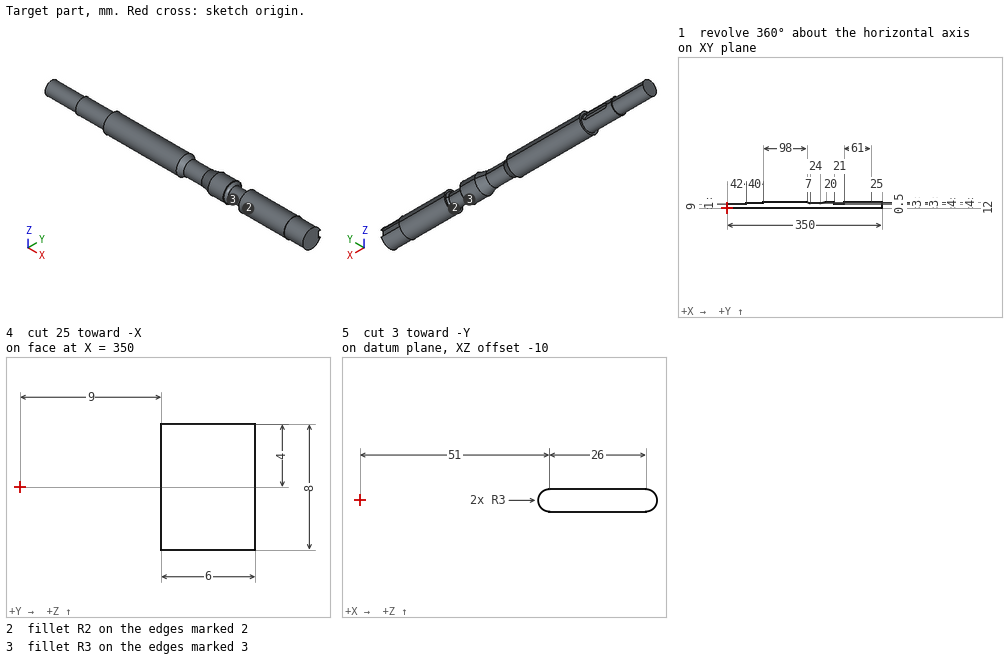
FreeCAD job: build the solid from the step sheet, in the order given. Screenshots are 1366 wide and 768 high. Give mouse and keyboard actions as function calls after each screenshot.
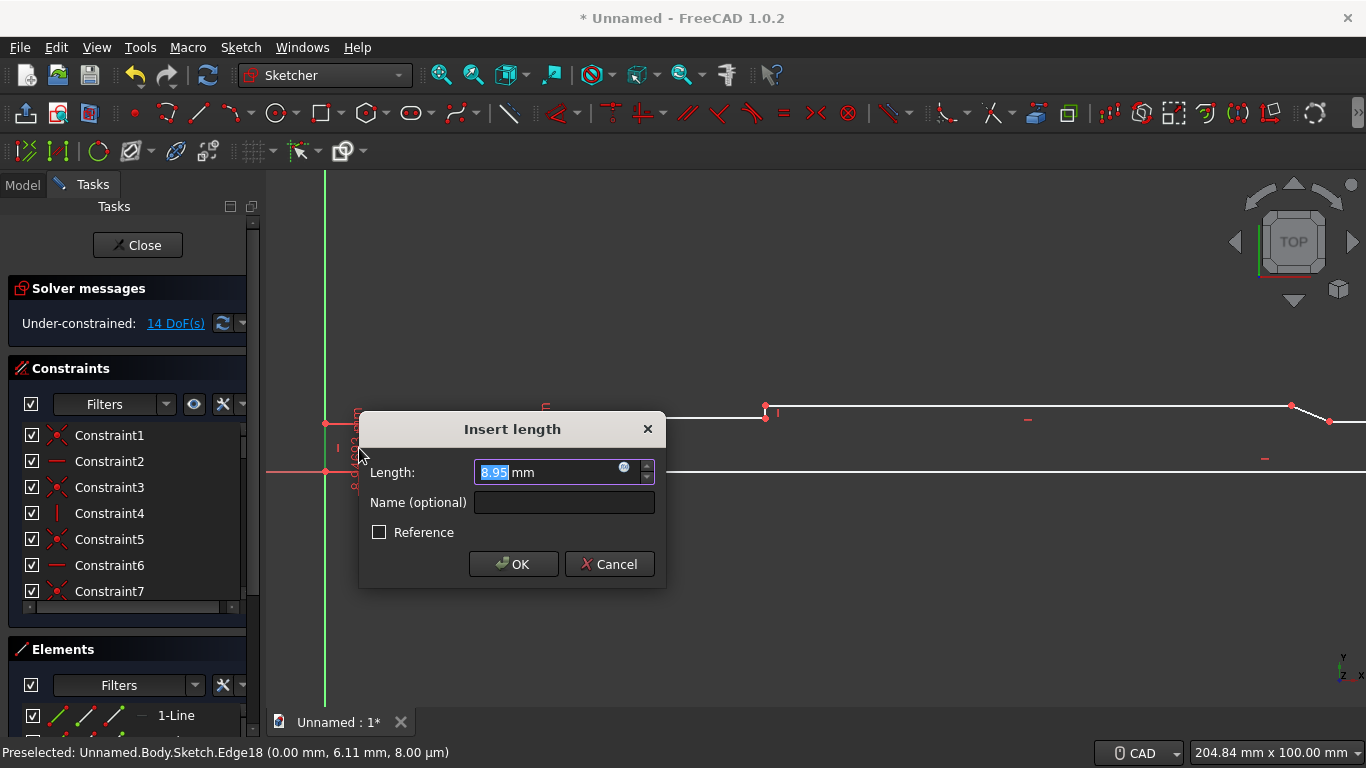
text(9)
key(Return)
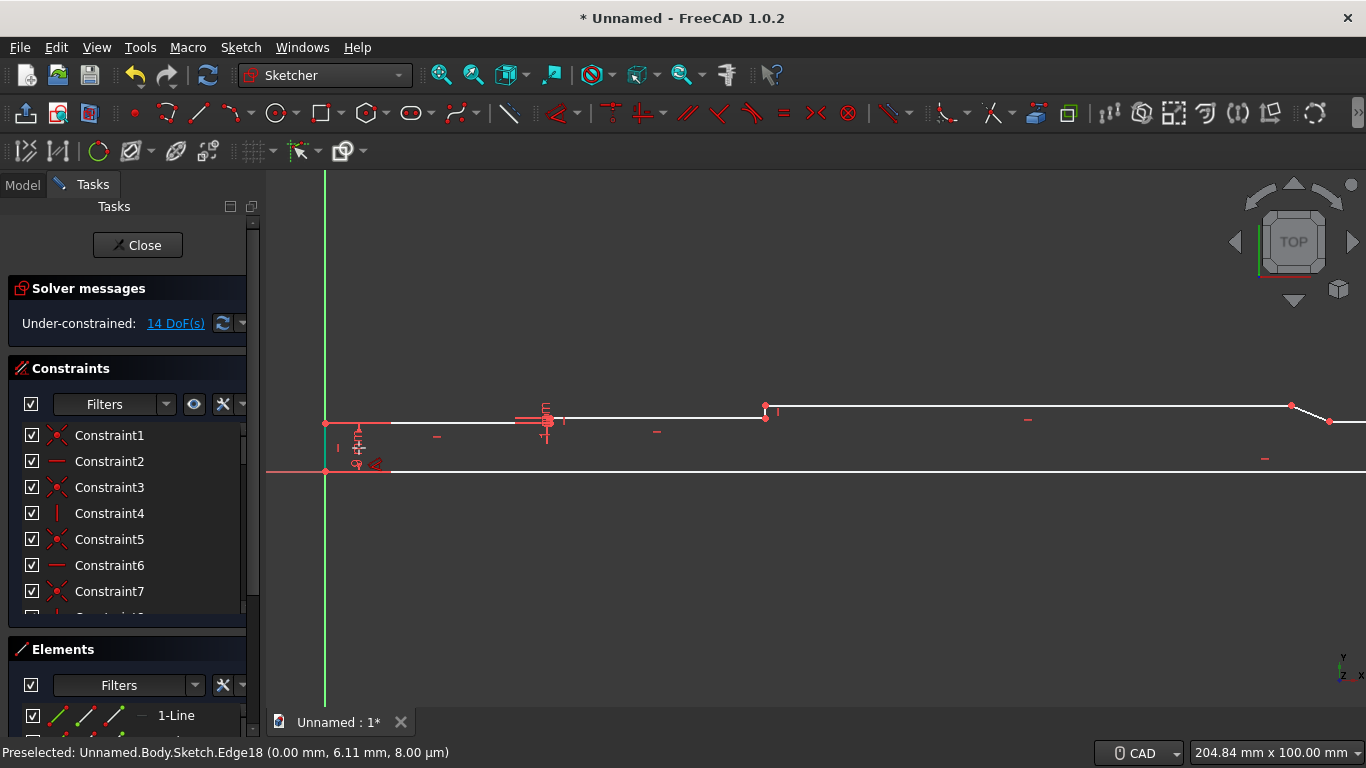
scroll(446, 439, down, 5)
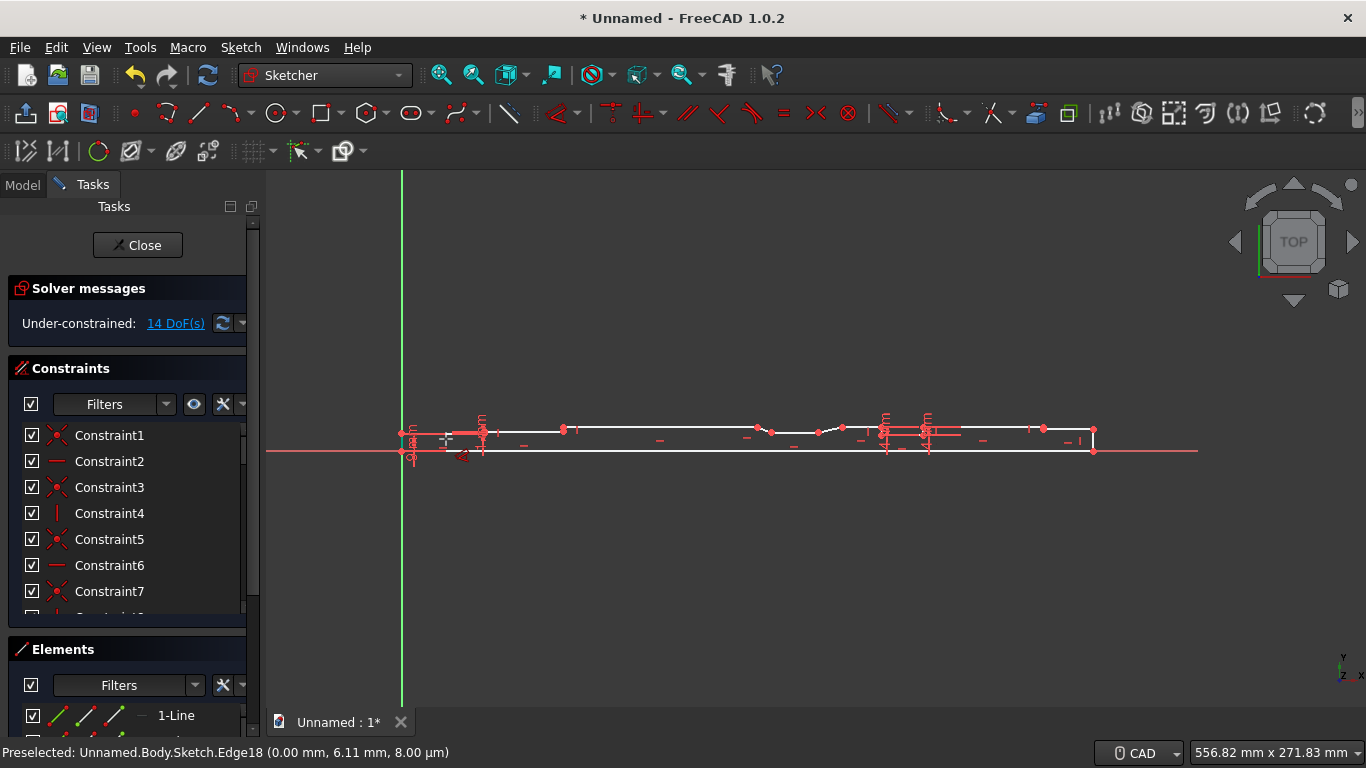
scroll(1093, 445, up, 4)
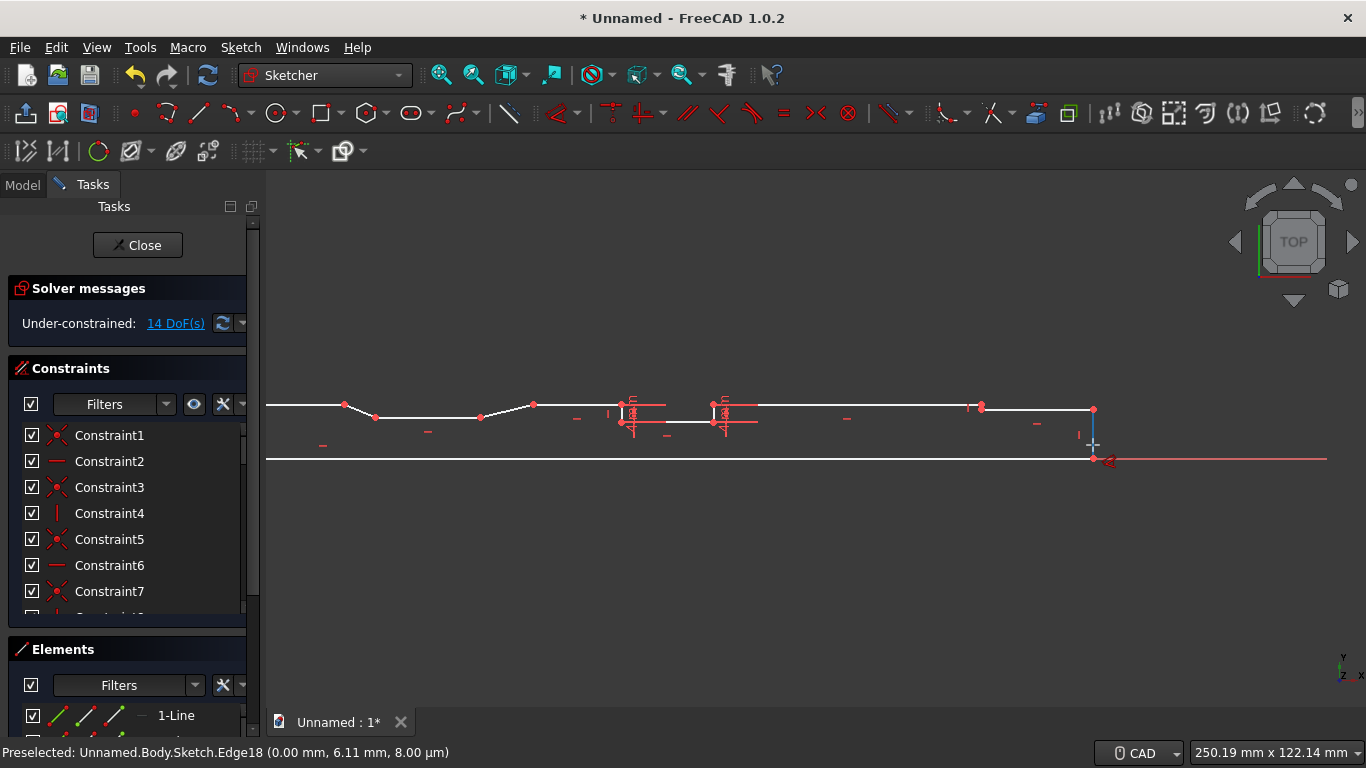
click(1093, 444)
click(1127, 434)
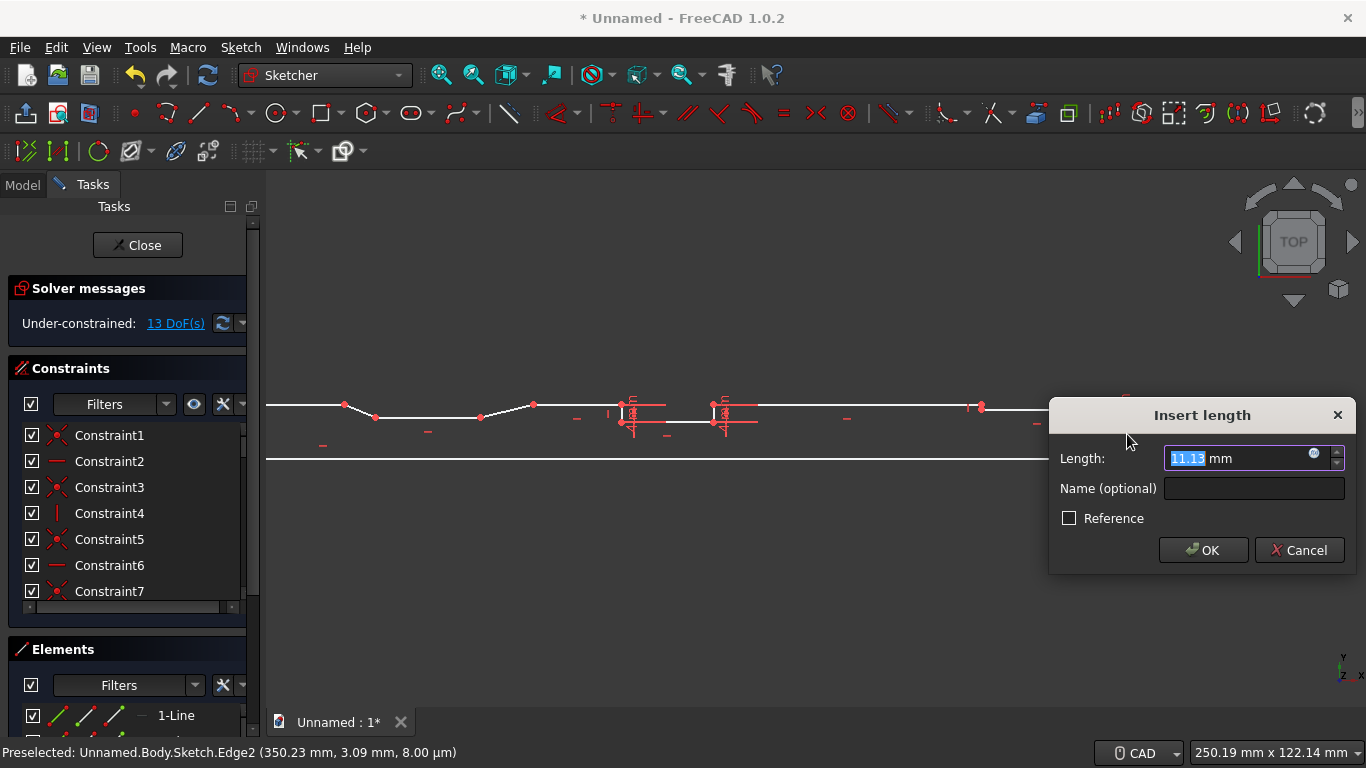
text(12)
key(Return)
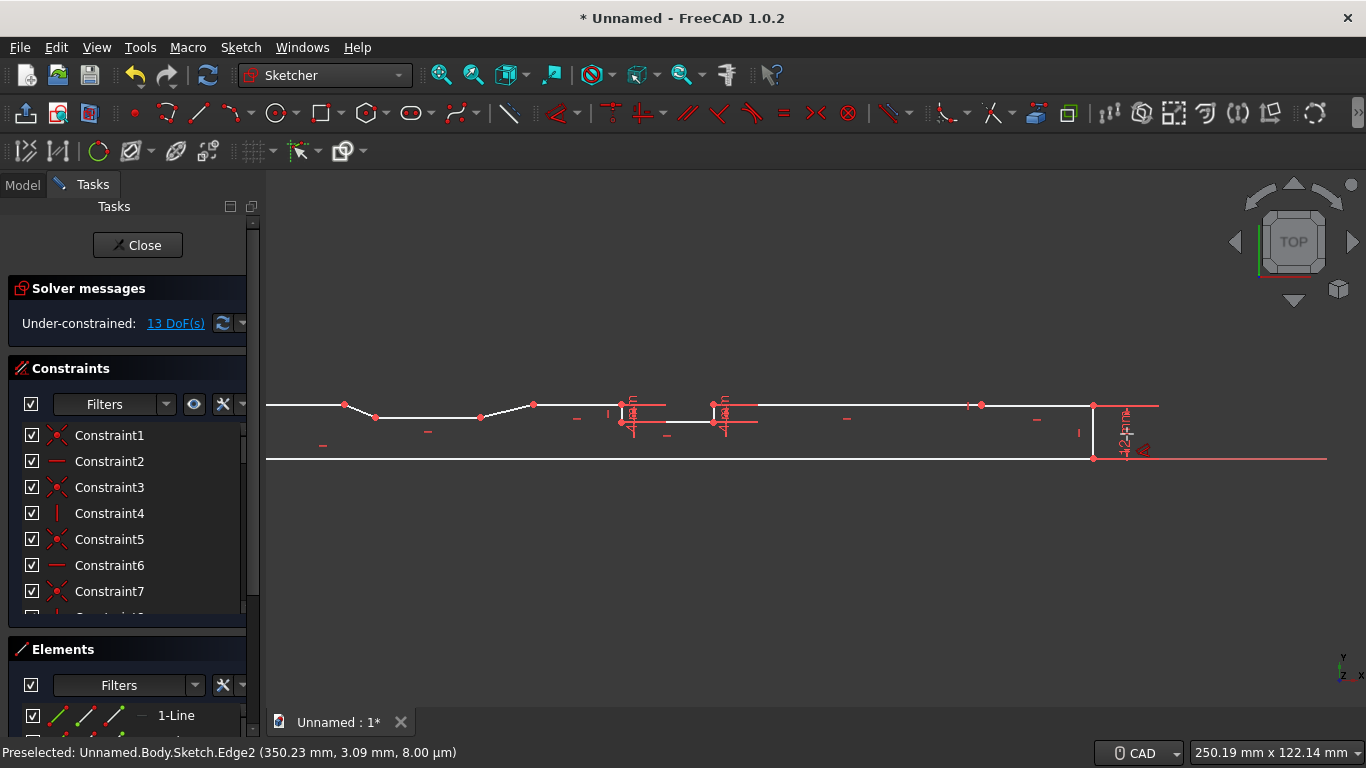
click(1060, 406)
click(1037, 372)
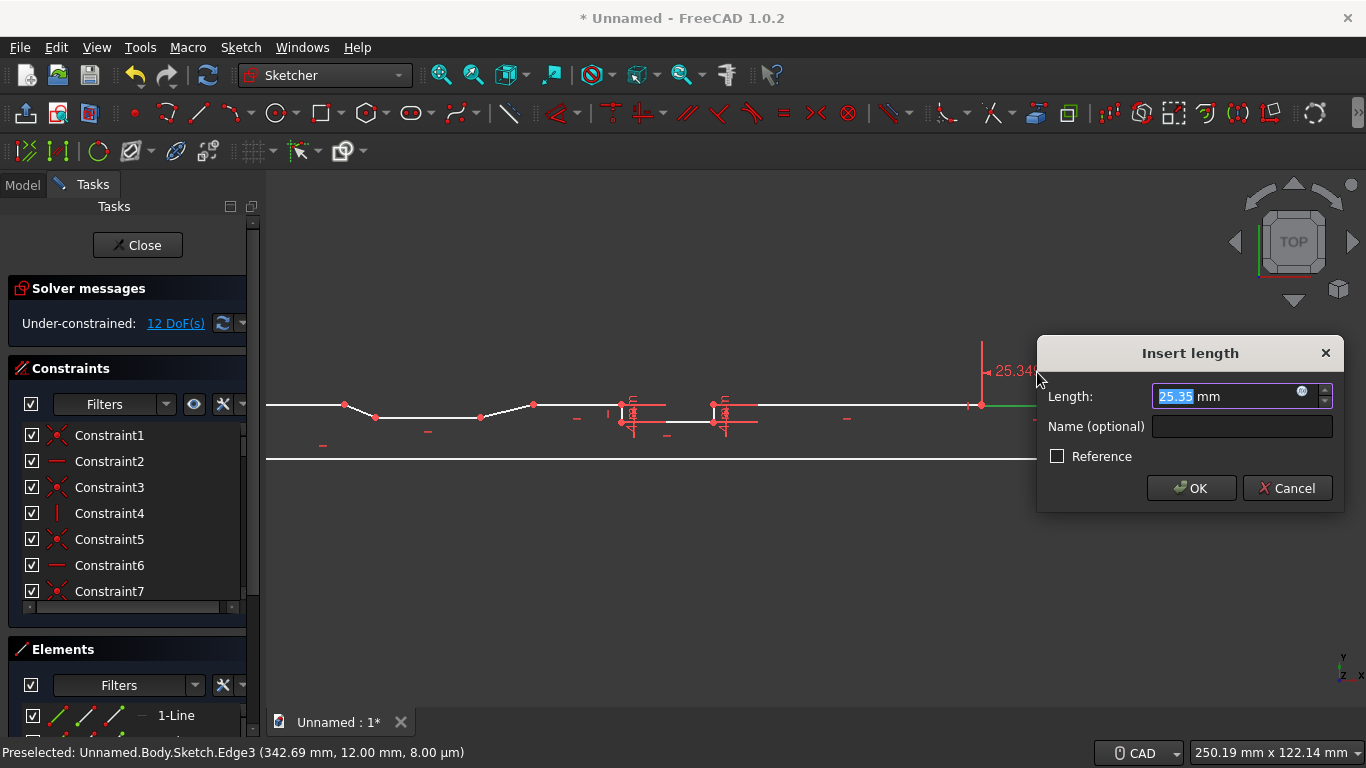
text(25)
key(Return)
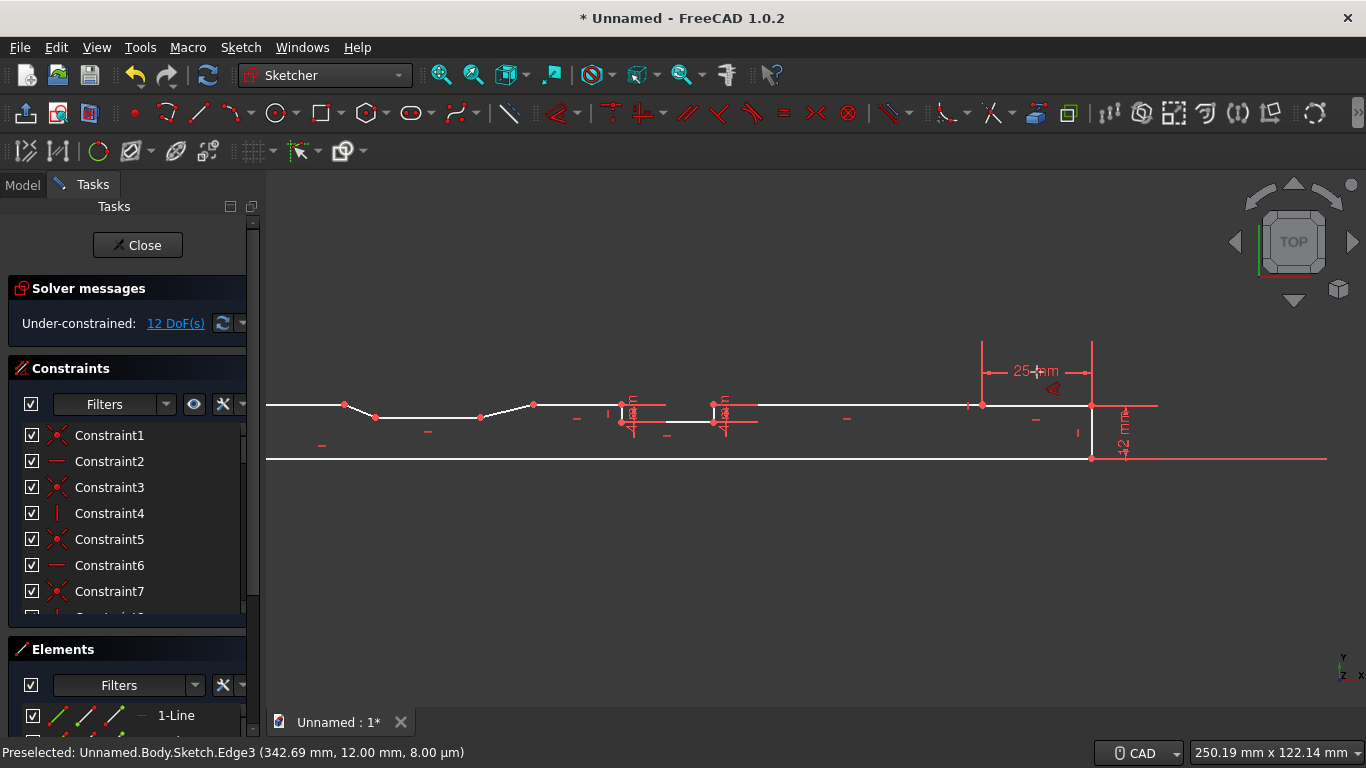
click(902, 405)
click(848, 371)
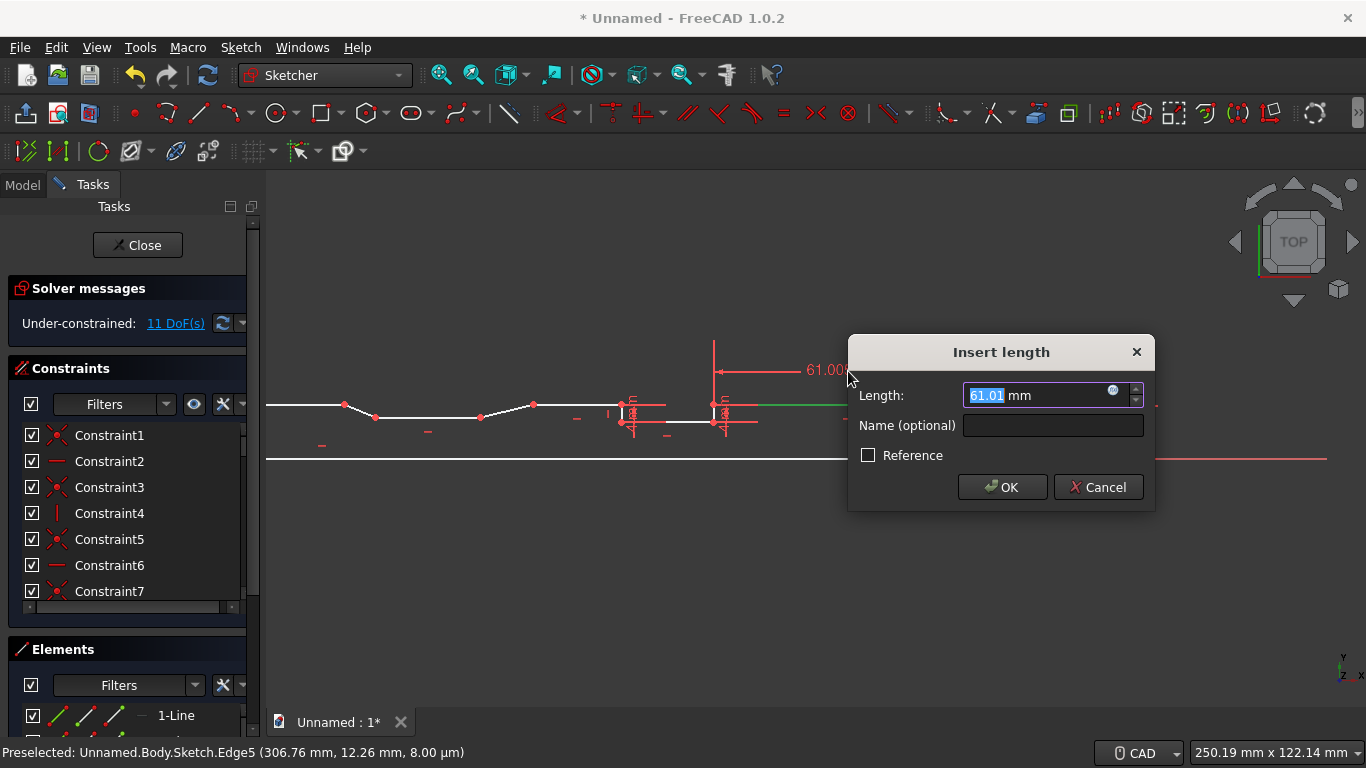
text(61)
key(Return)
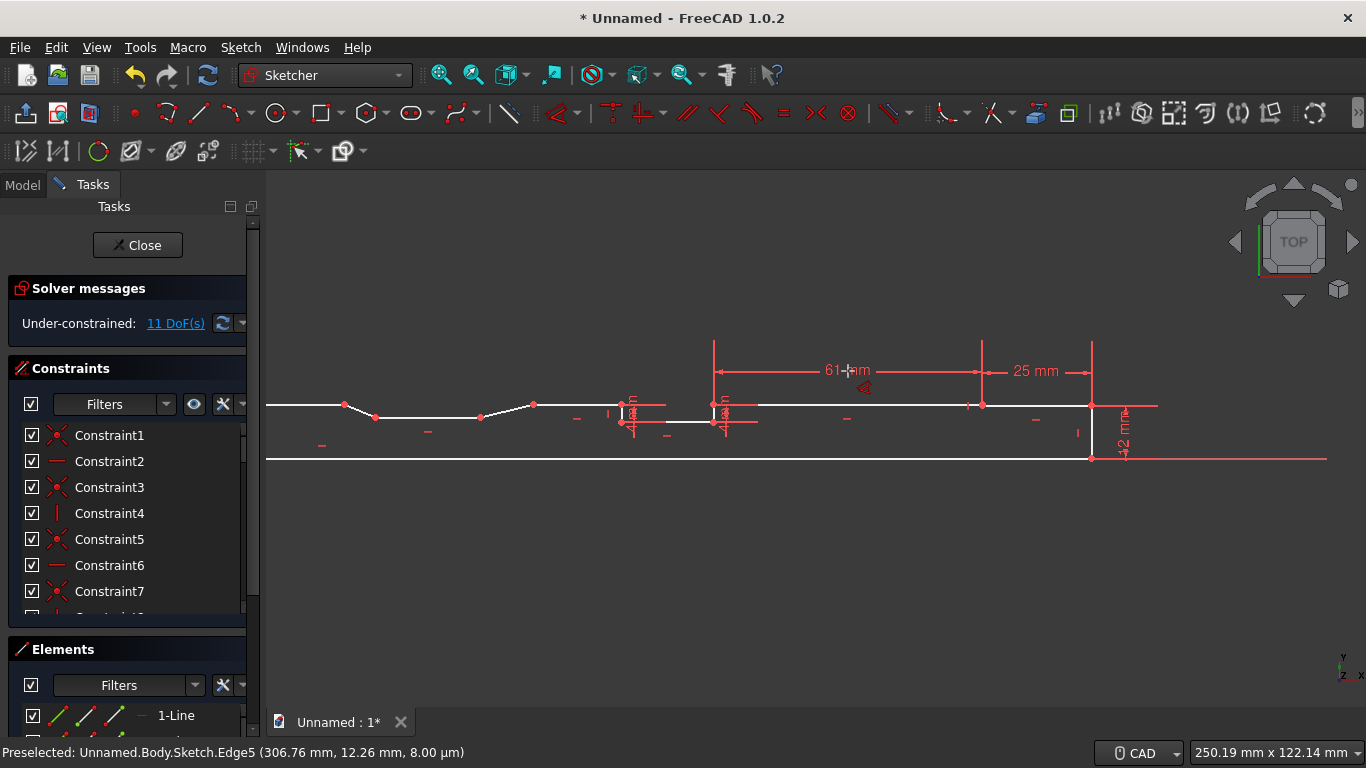
click(686, 422)
click(668, 388)